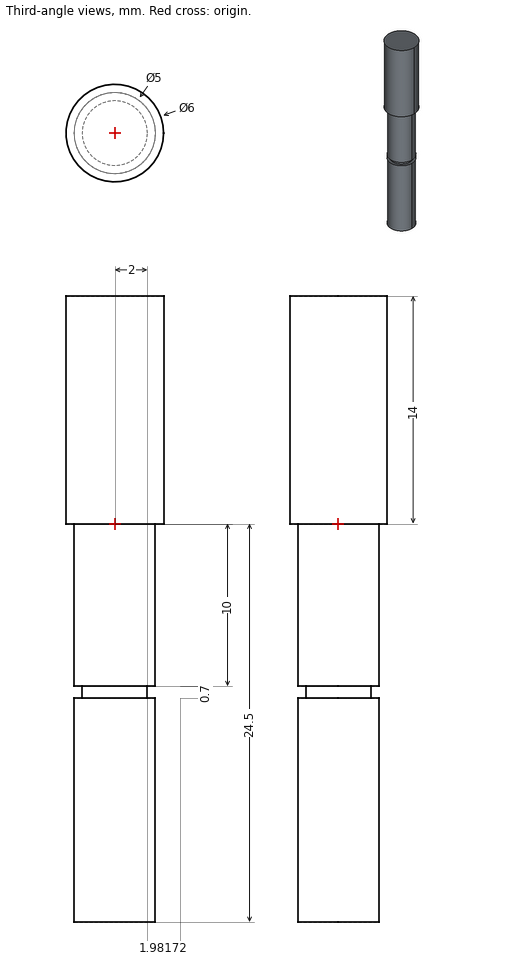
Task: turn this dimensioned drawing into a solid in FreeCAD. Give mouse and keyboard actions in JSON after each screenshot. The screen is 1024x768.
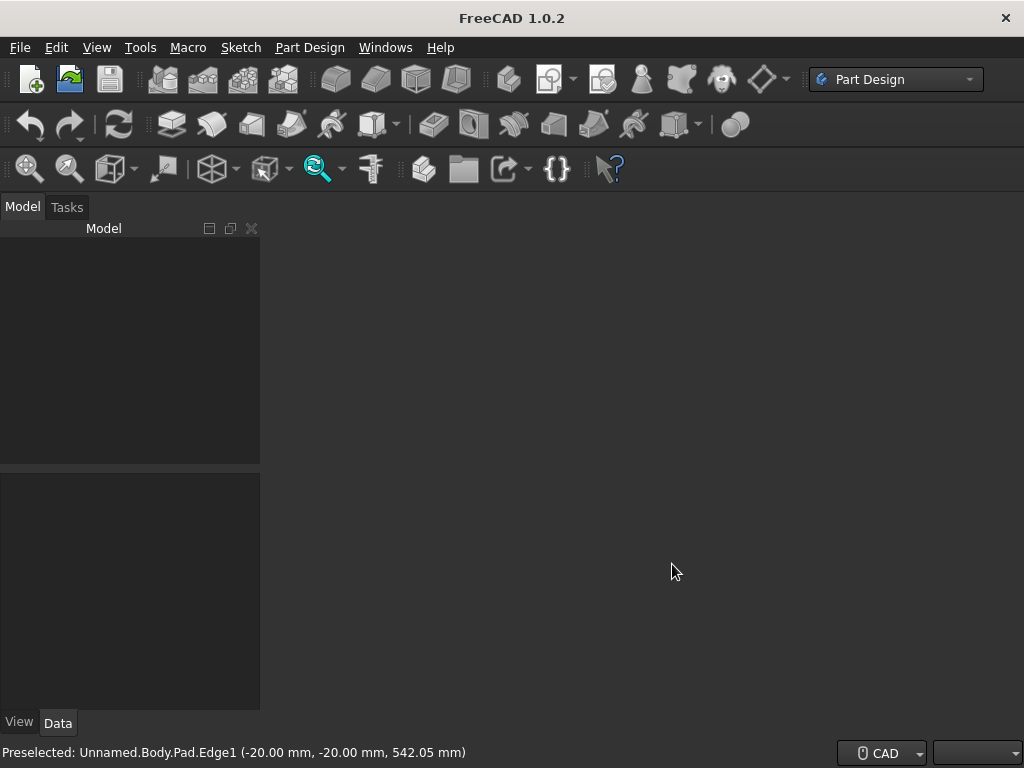
{"action": "left_click", "coordinate": [30, 80]}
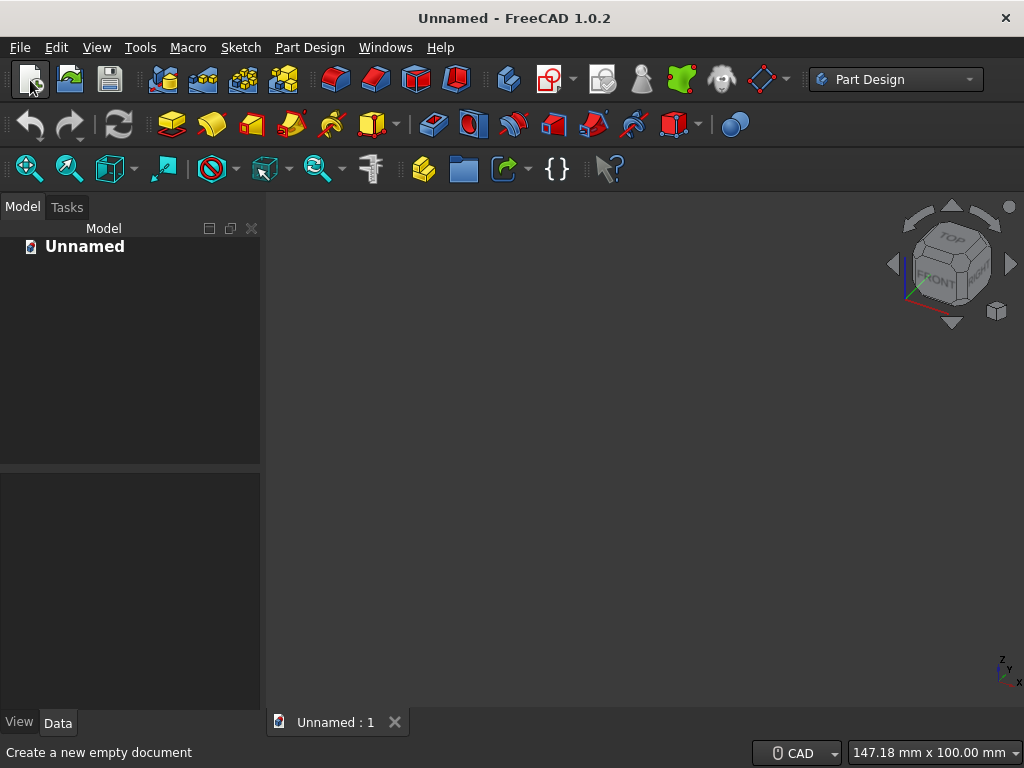
{"action": "left_click", "coordinate": [550, 80]}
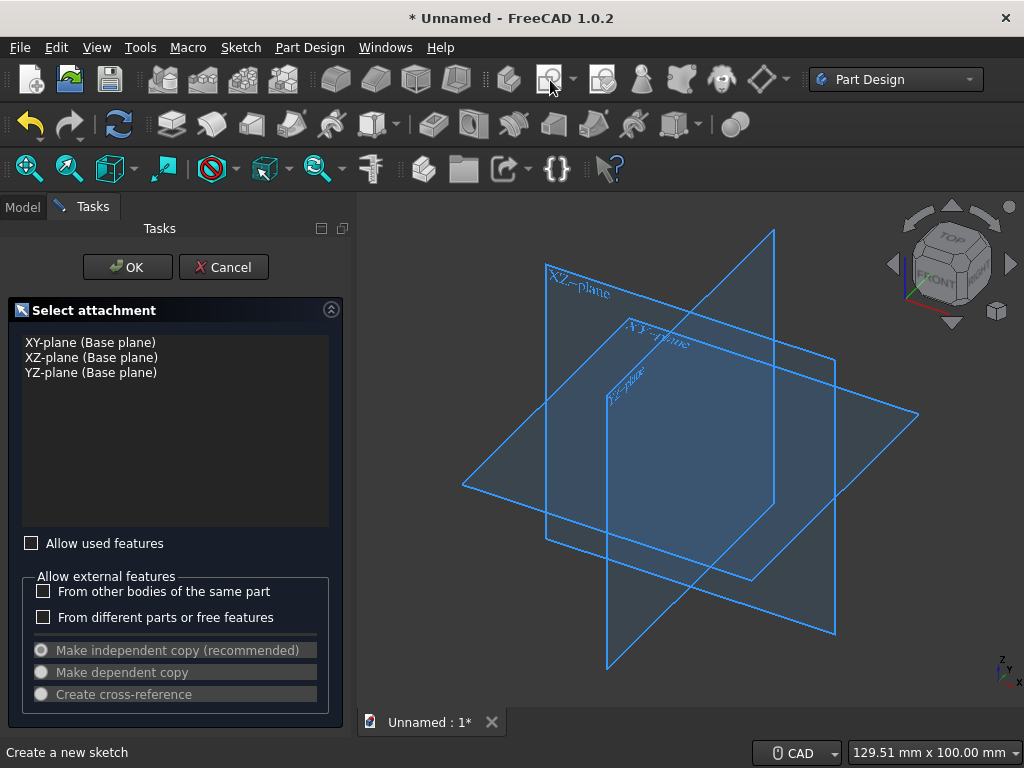
{"action": "left_click", "coordinate": [82, 342]}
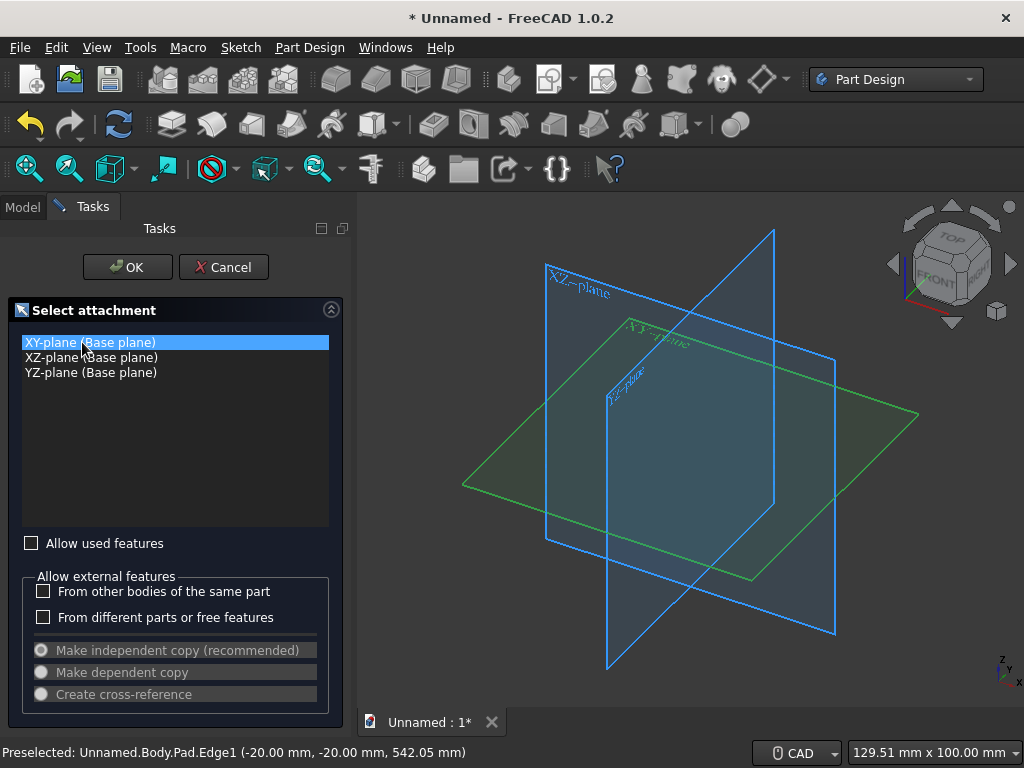
{"action": "left_click", "coordinate": [128, 267]}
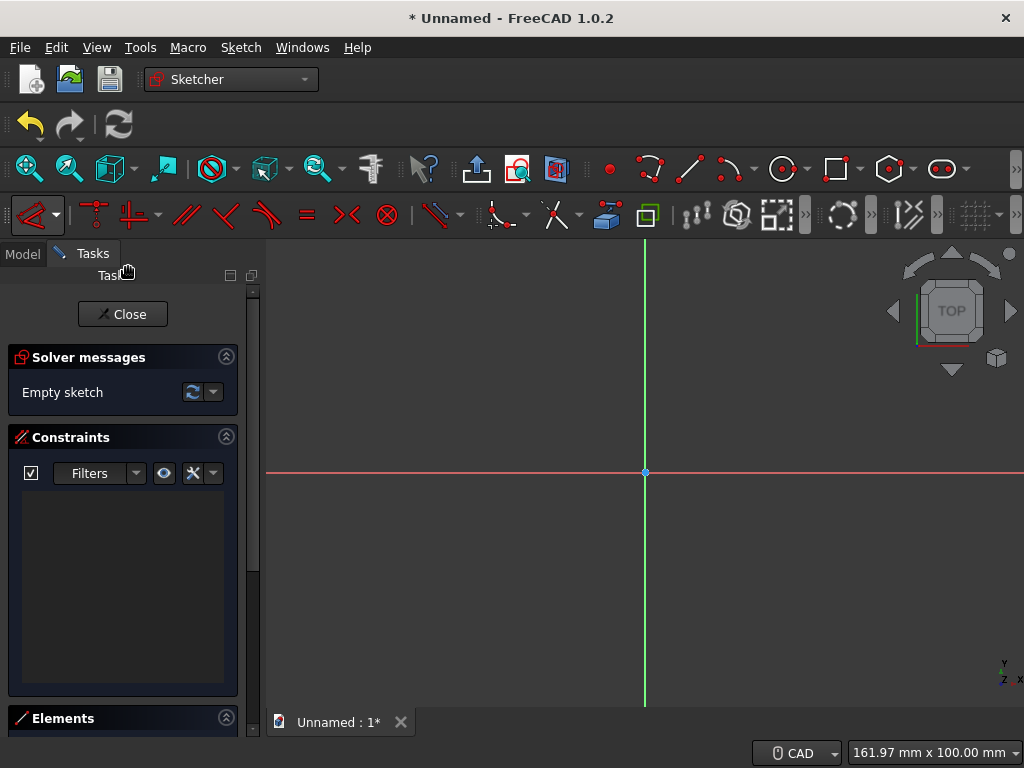
{"action": "scroll", "coordinate": [652, 473], "scroll_direction": "up", "scroll_amount": 12}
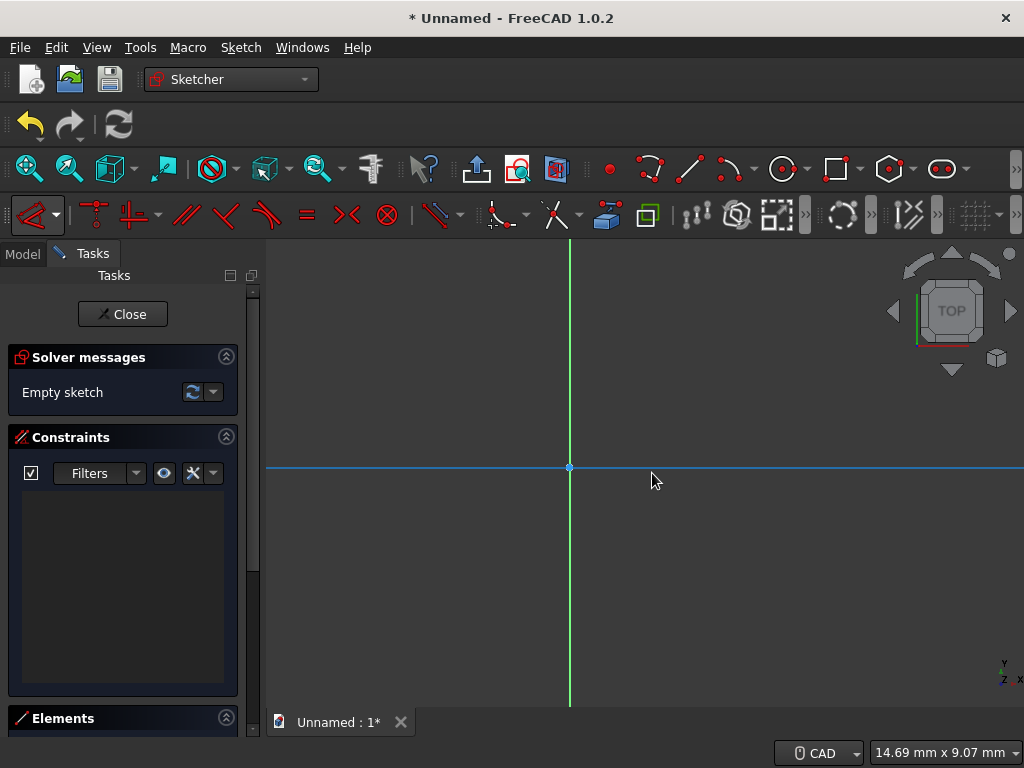
{"action": "left_click", "coordinate": [784, 170]}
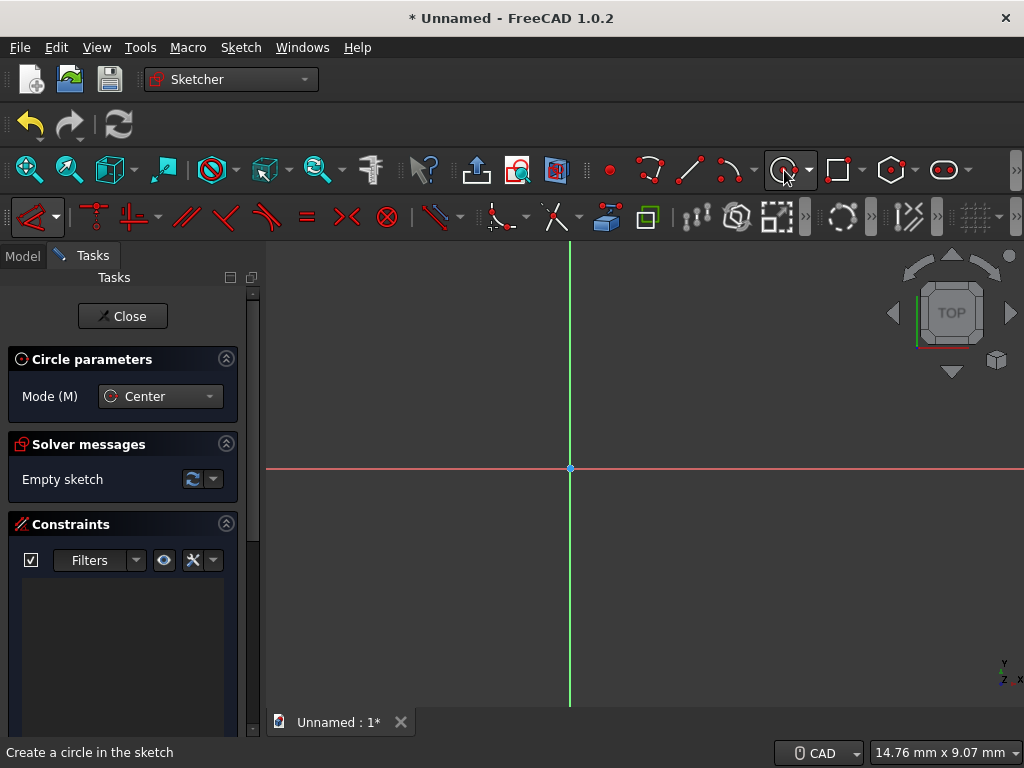
{"action": "left_click", "coordinate": [570, 469]}
{"action": "mouse_move", "coordinate": [679, 360]}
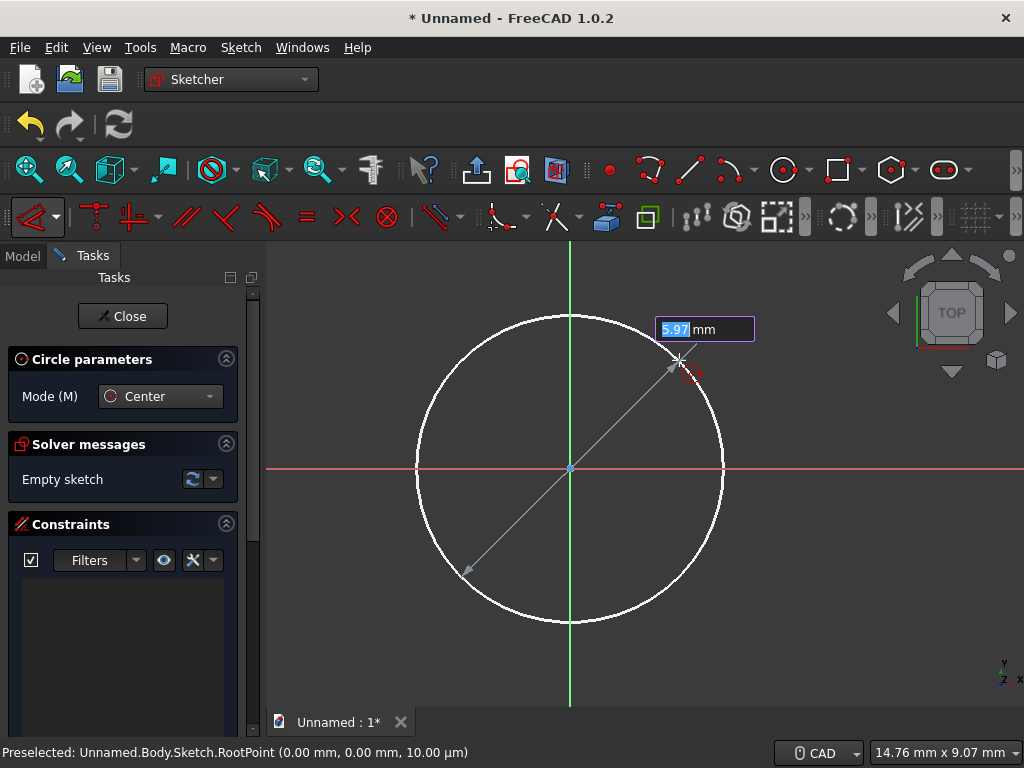
{"action": "type", "text": "6"}
{"action": "key", "text": "Return"}
{"action": "key", "text": "Escape"}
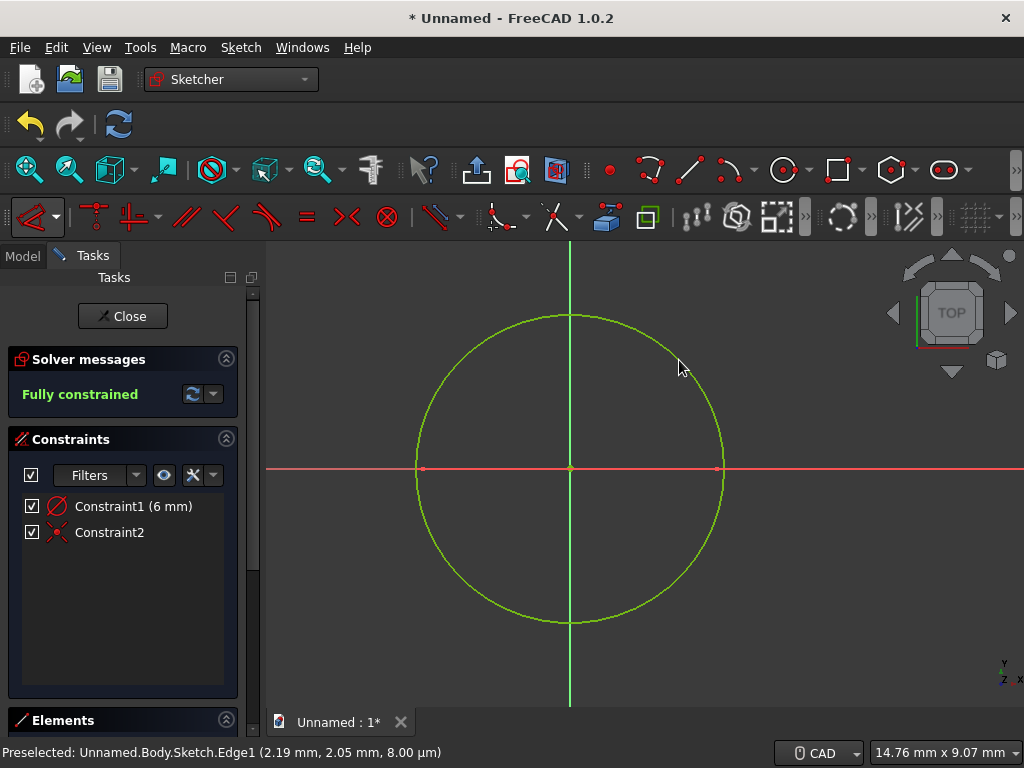
{"action": "left_click", "coordinate": [123, 316]}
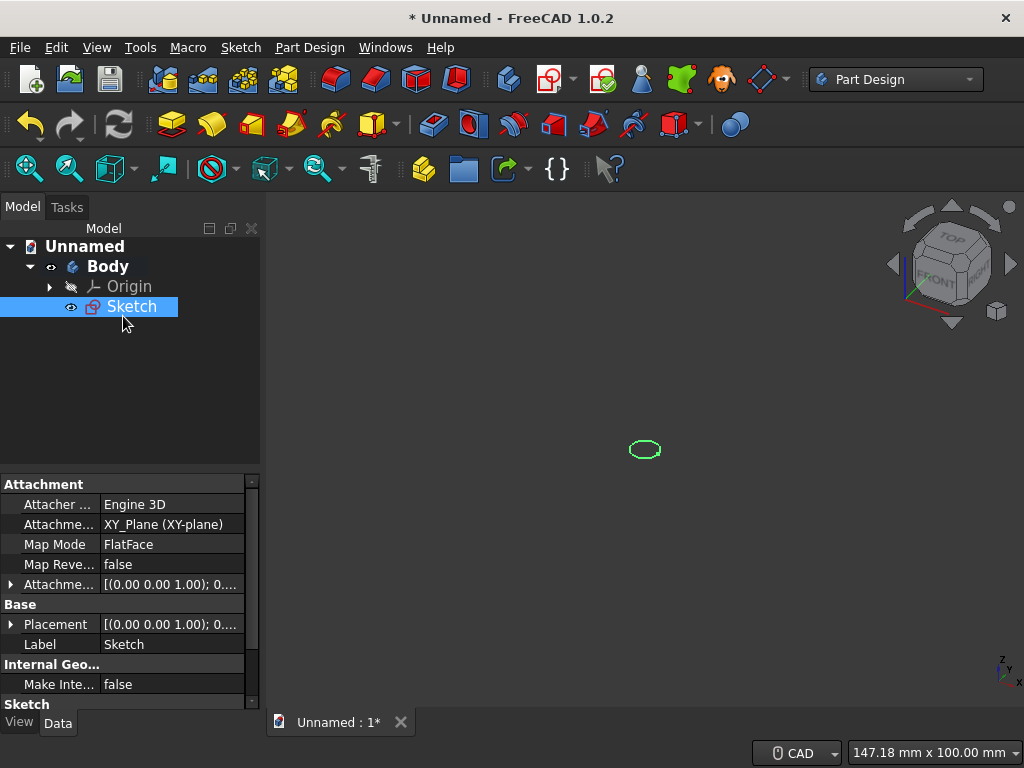
{"action": "left_click", "coordinate": [172, 124]}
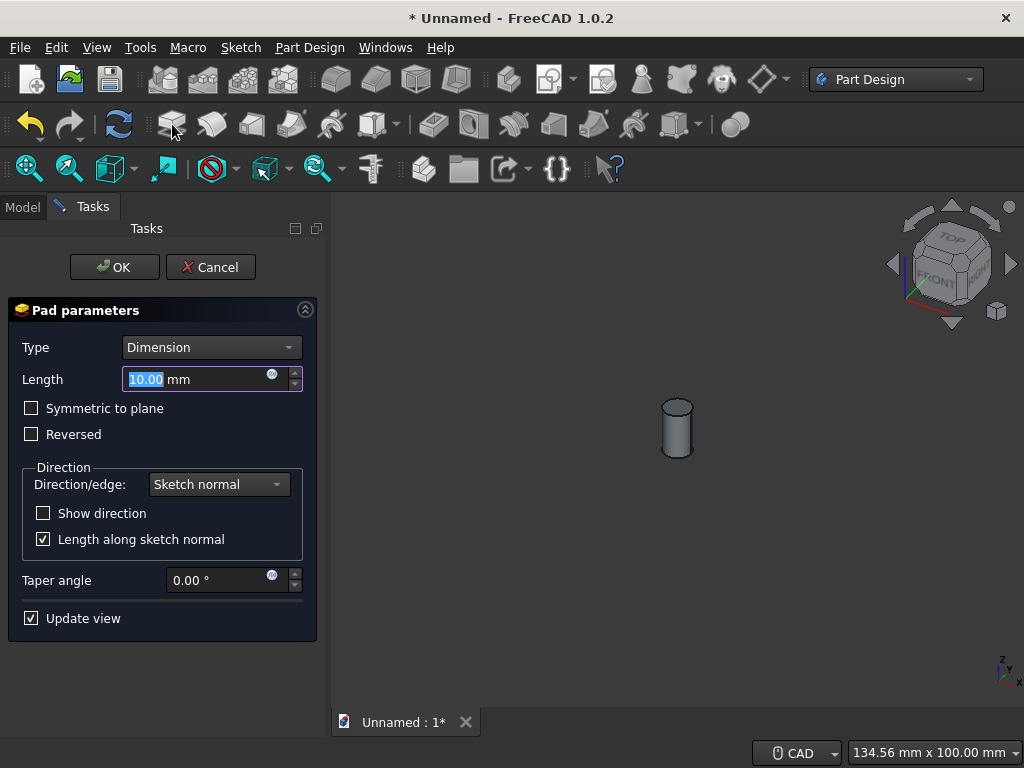
{"action": "type", "text": "14"}
{"action": "key", "text": "Tab"}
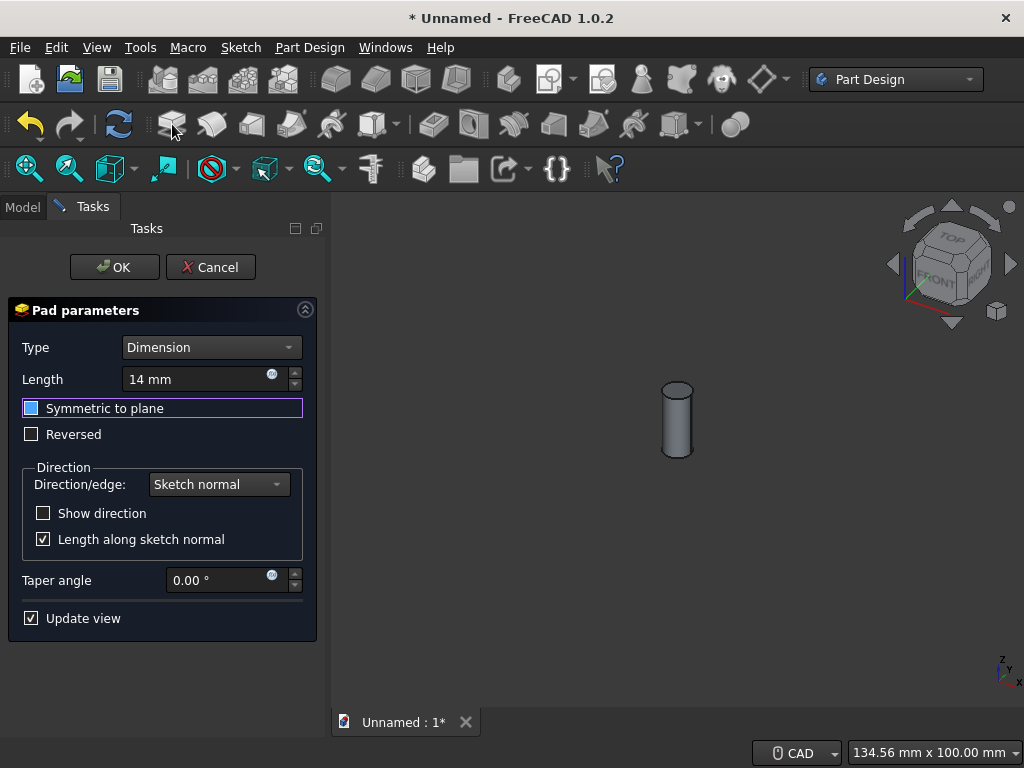
{"action": "left_click", "coordinate": [115, 267]}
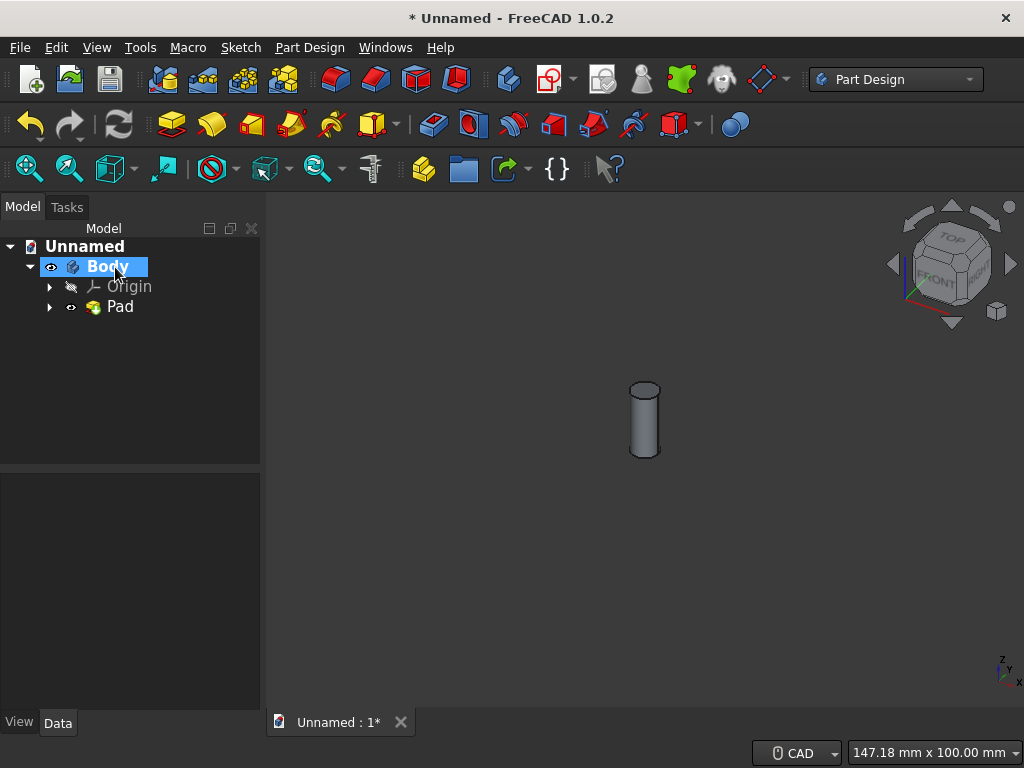
{"action": "key", "text": "v f"}